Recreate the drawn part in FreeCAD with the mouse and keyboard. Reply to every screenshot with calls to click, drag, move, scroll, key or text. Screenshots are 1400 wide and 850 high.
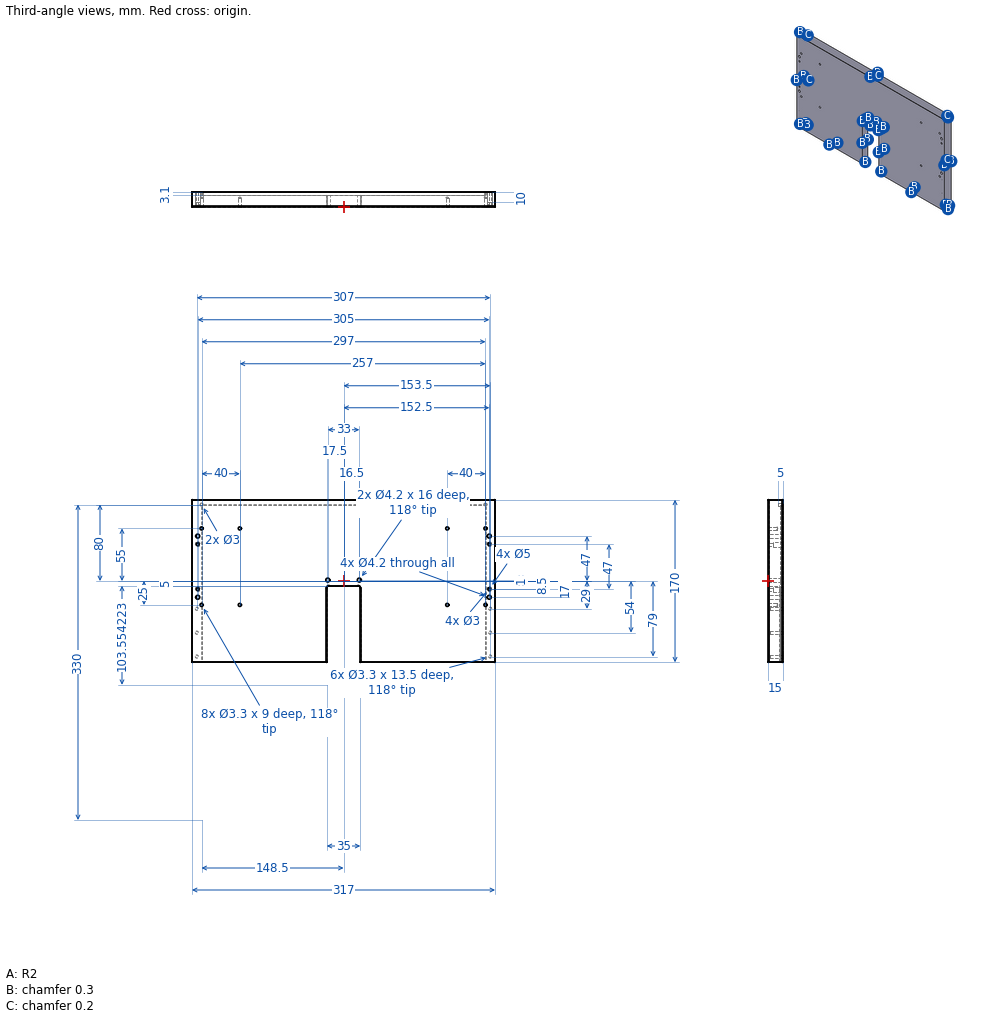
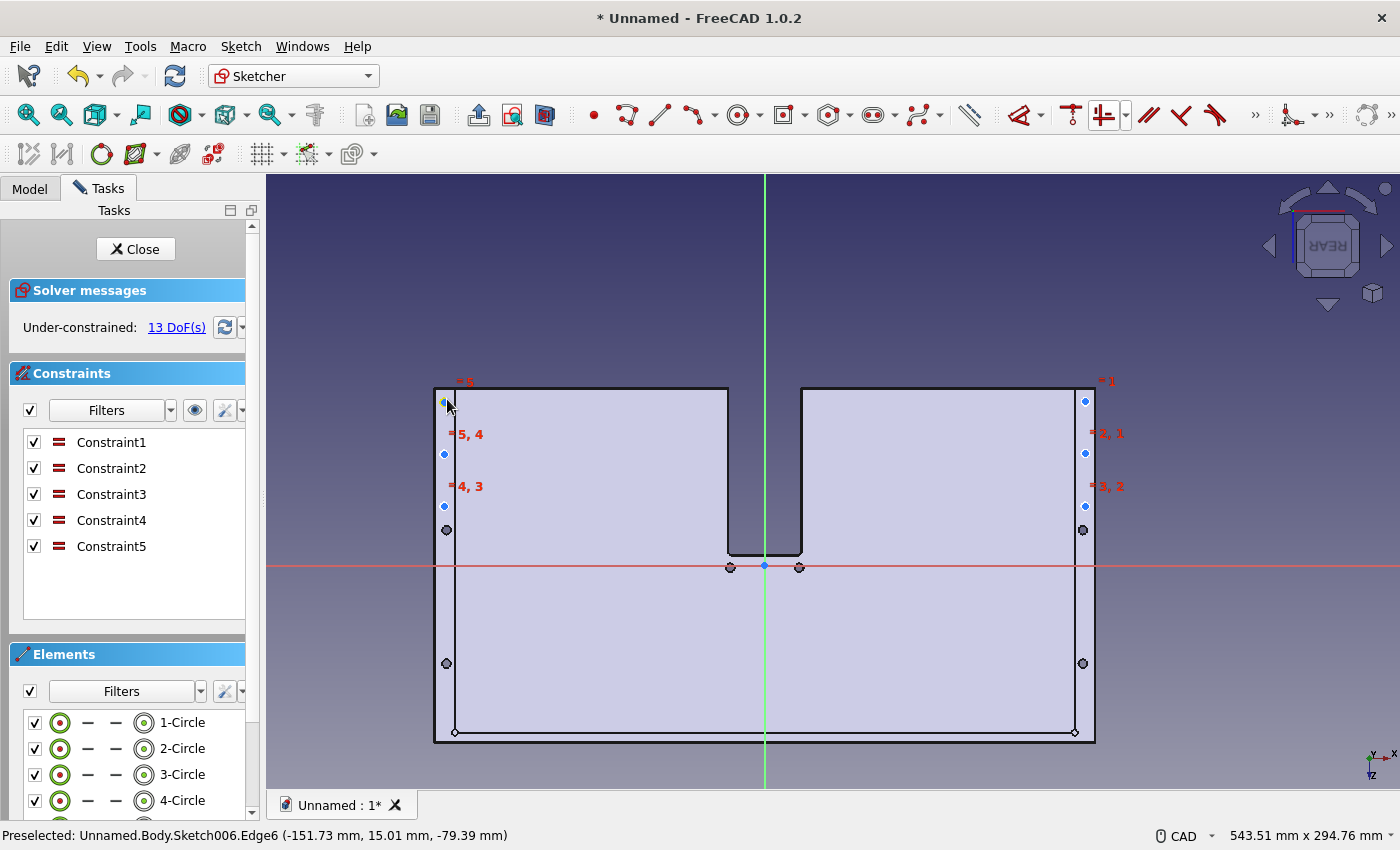
click(1085, 402)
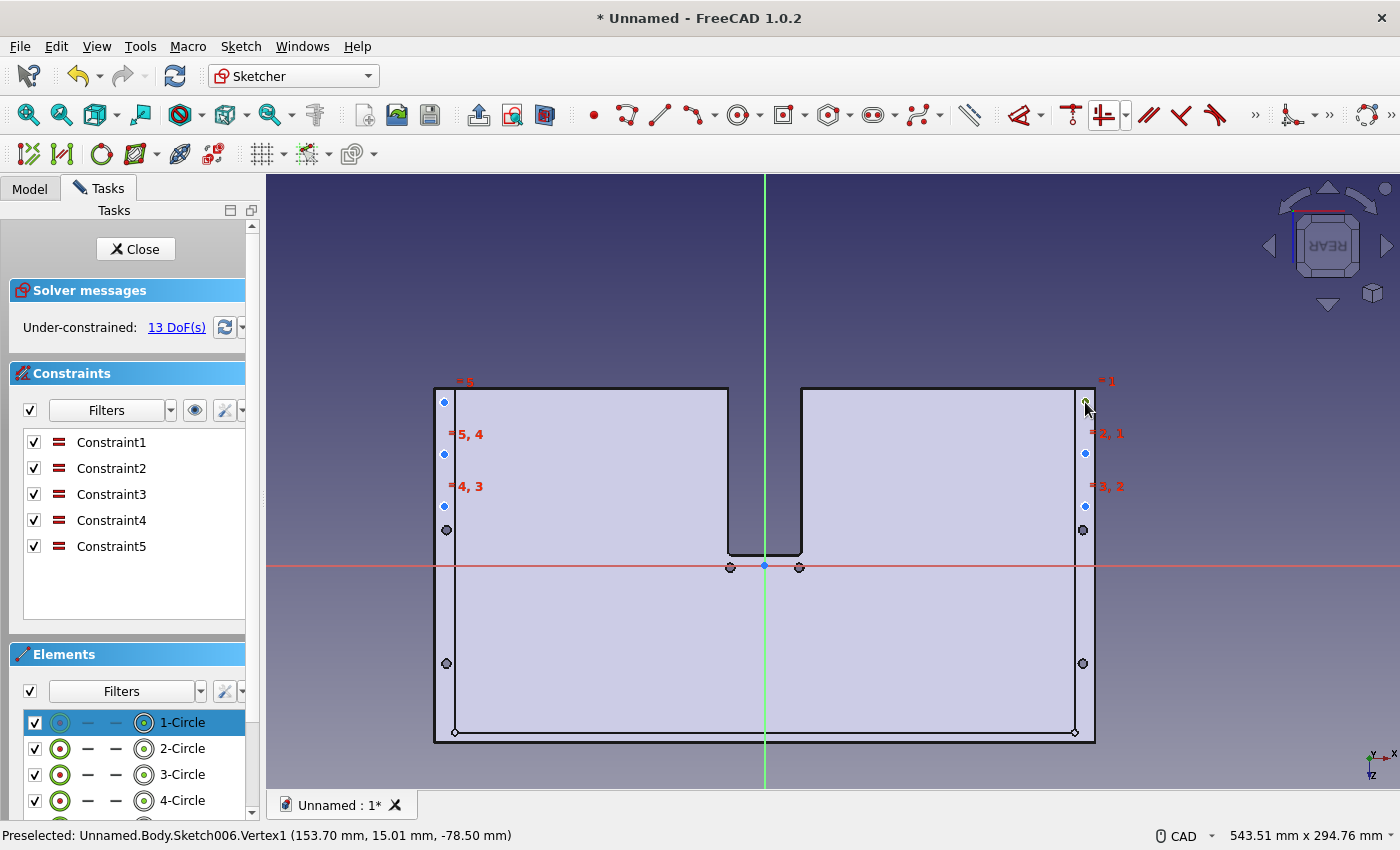
click(1085, 453)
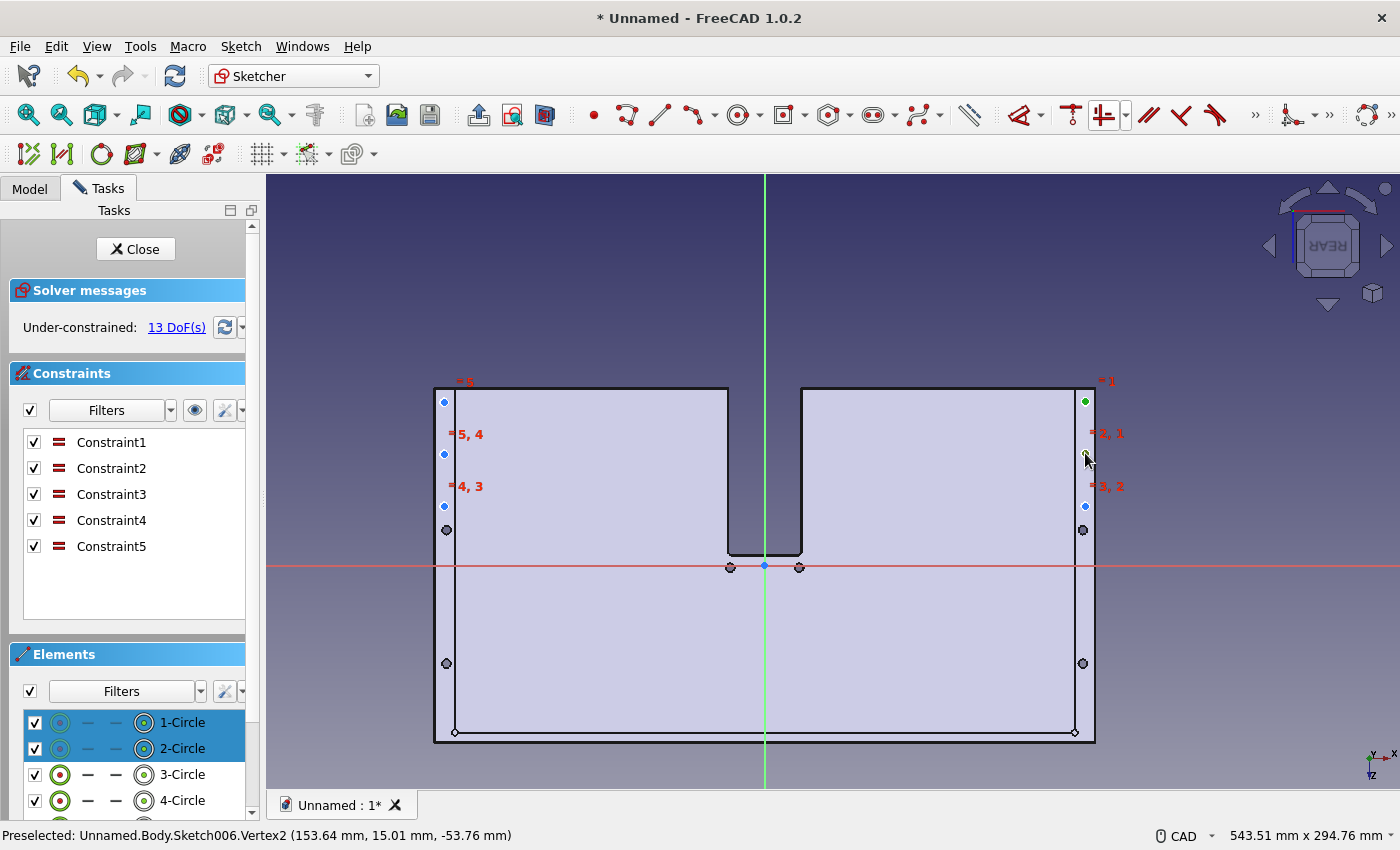
key(v)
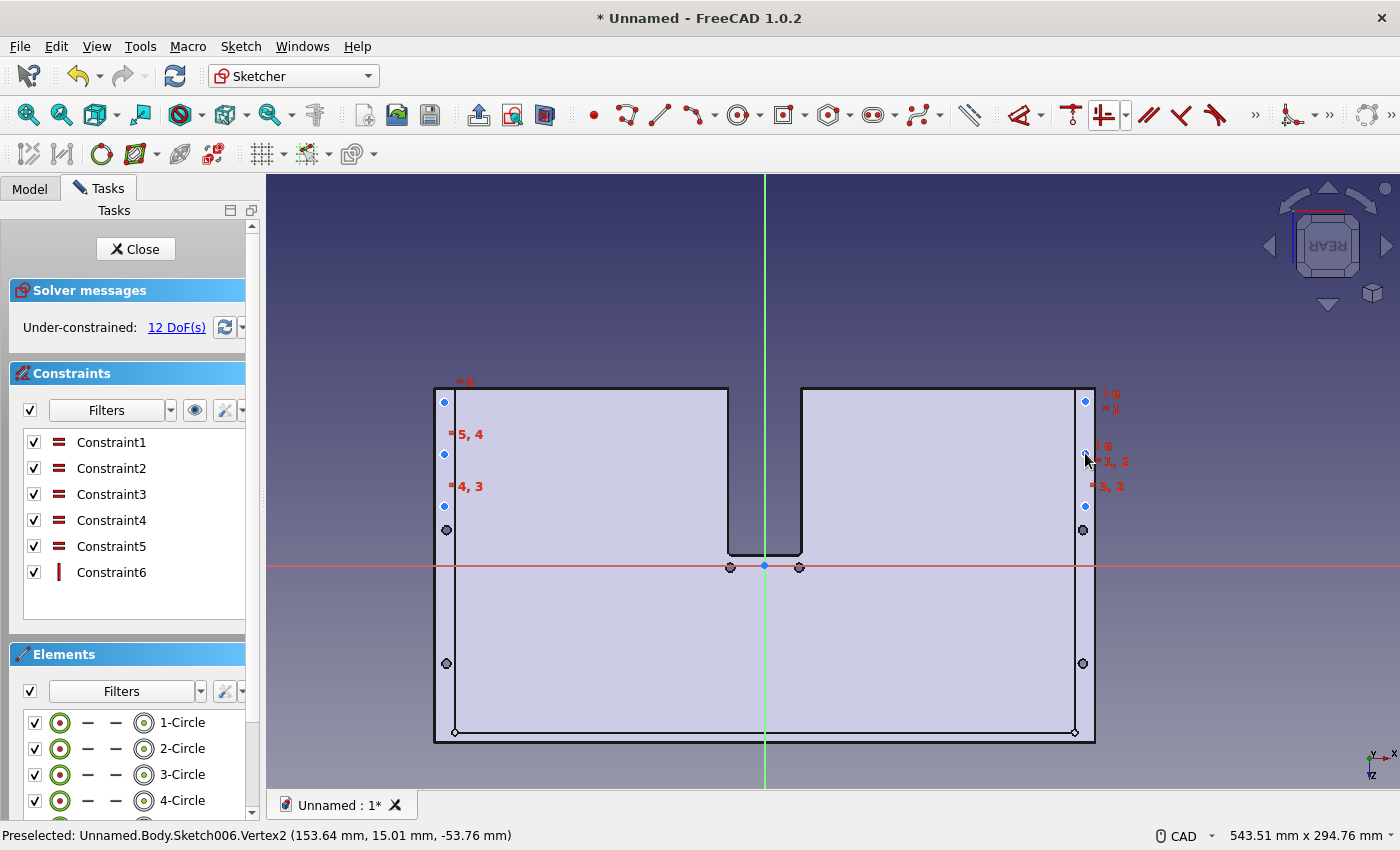
click(1085, 453)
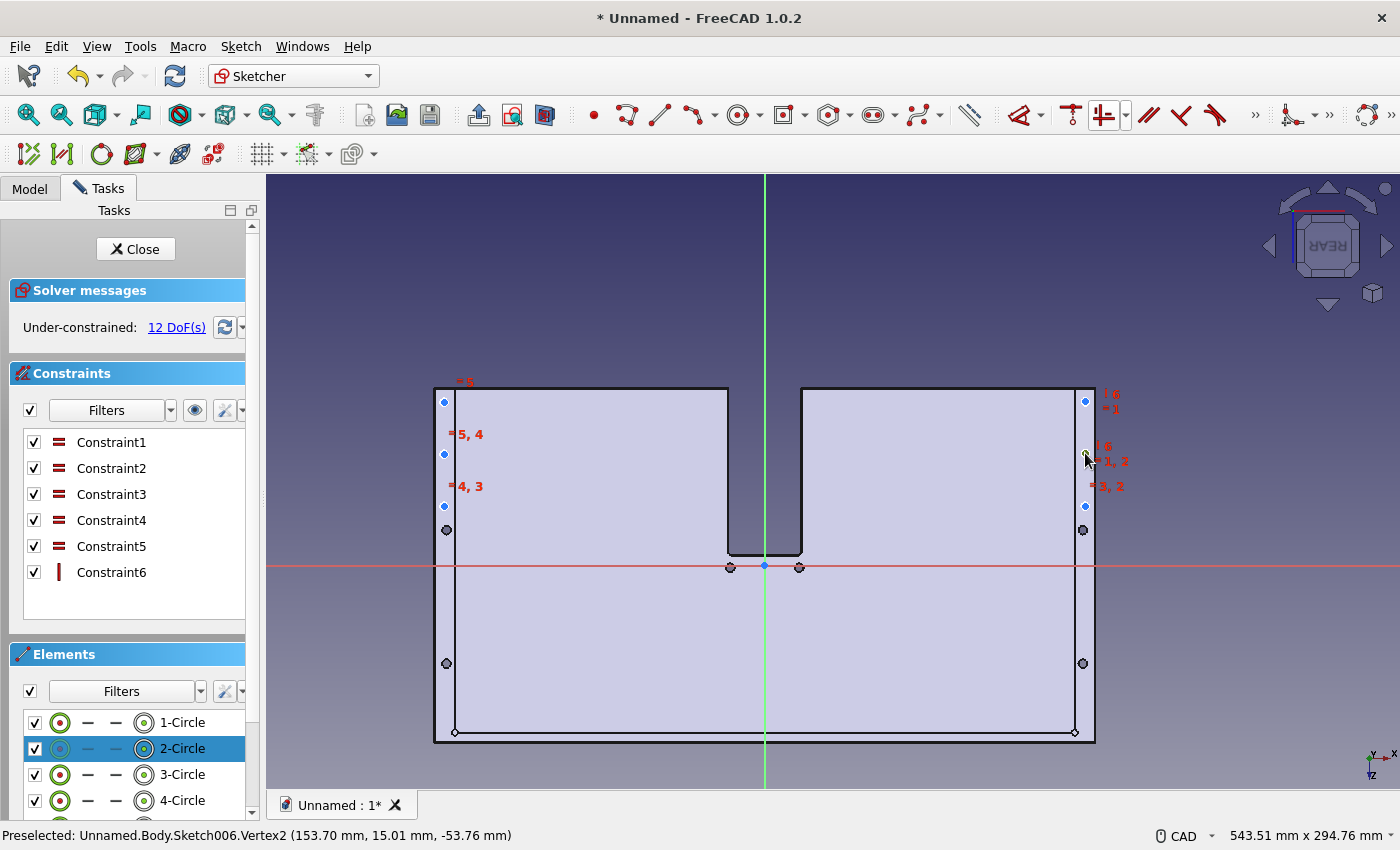
click(1085, 506)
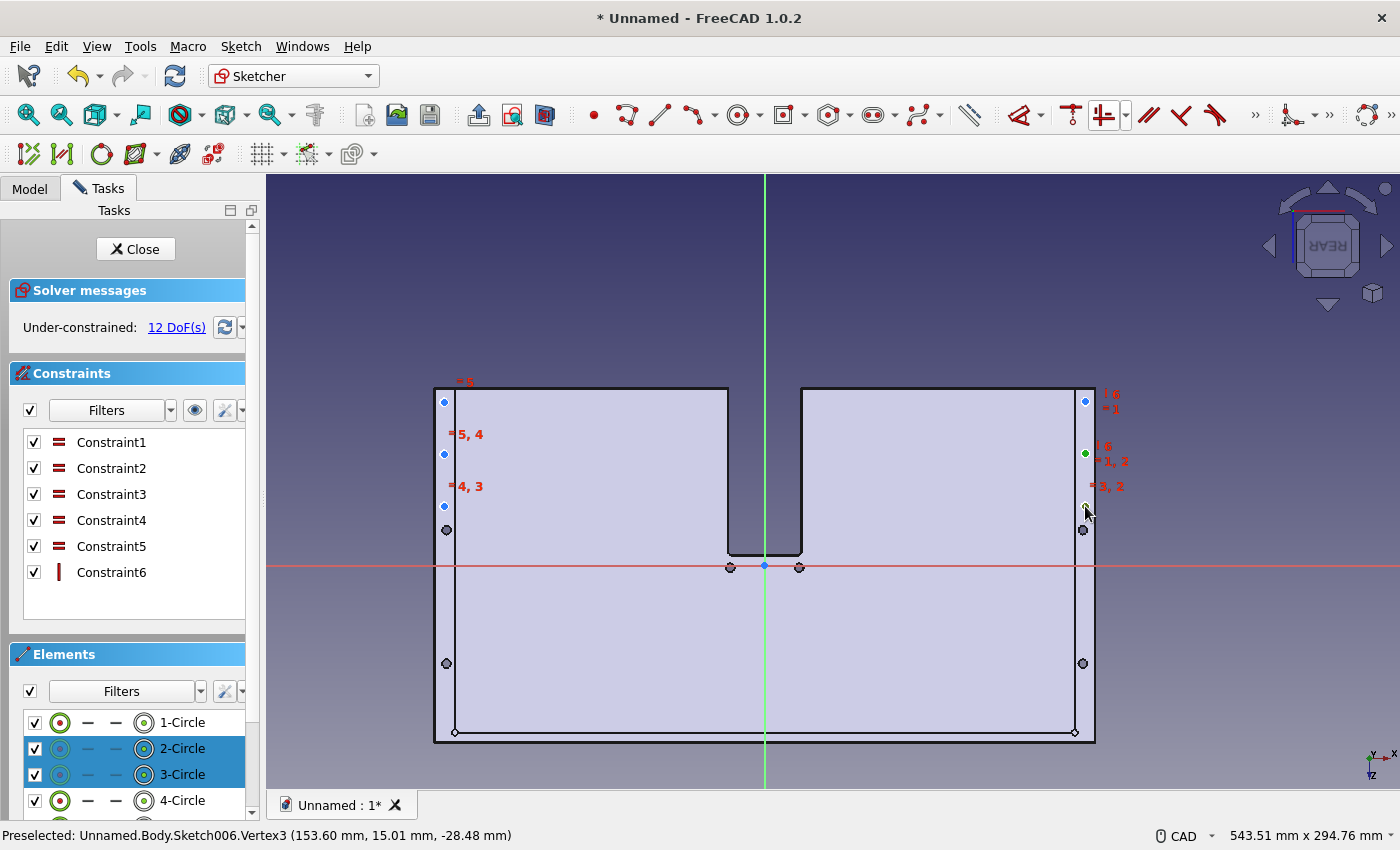
click(1126, 116)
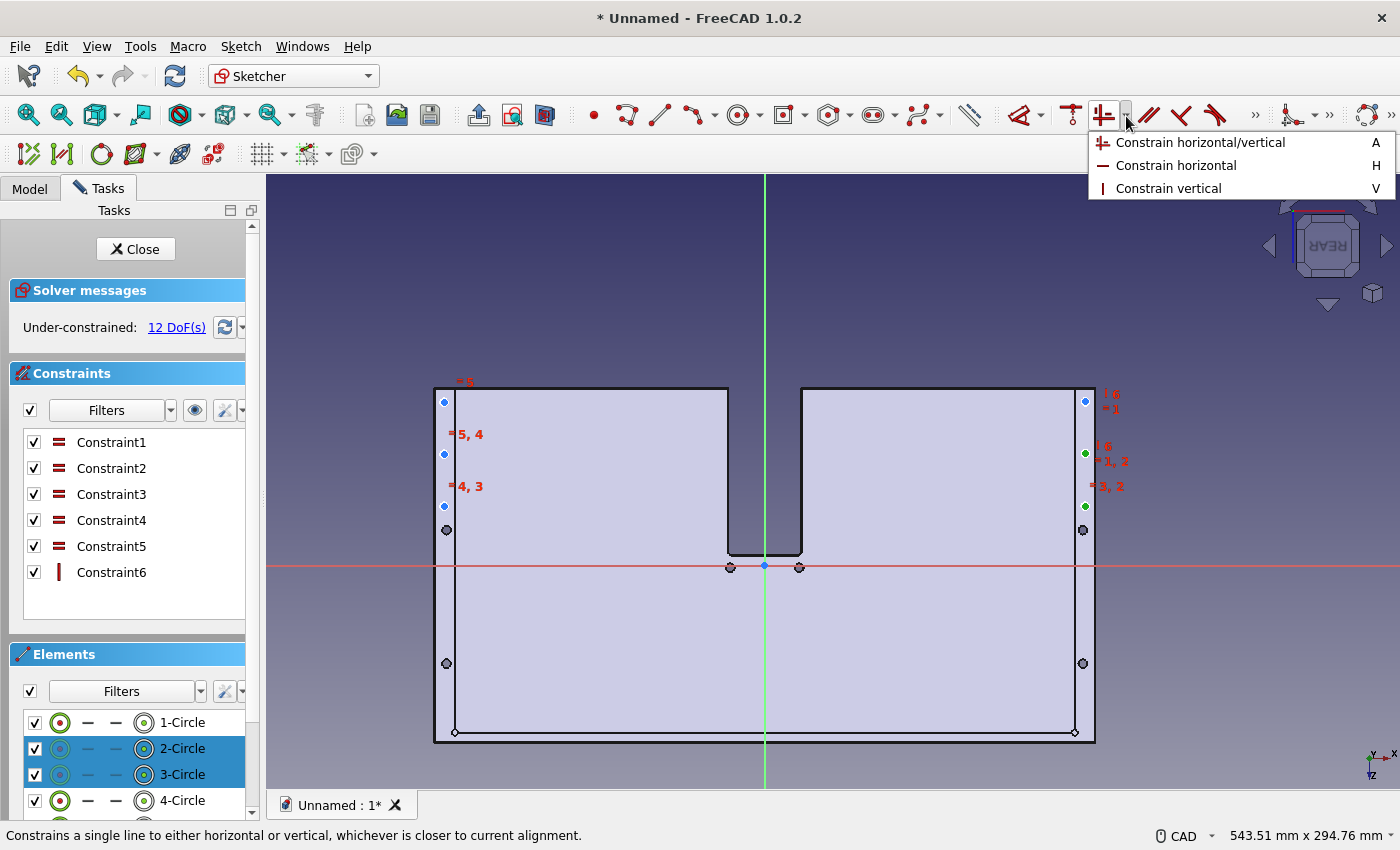
click(1242, 188)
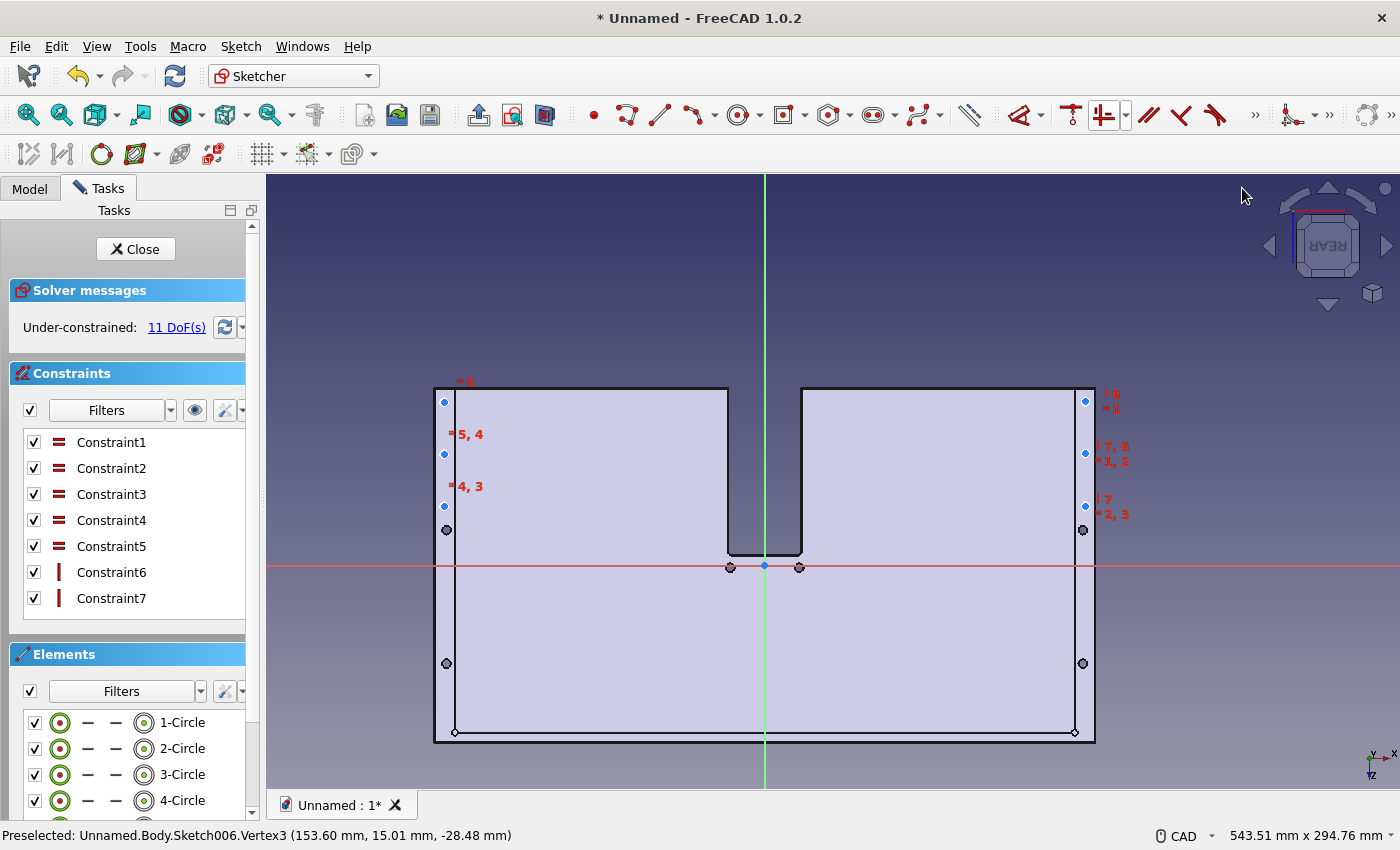
click(1085, 506)